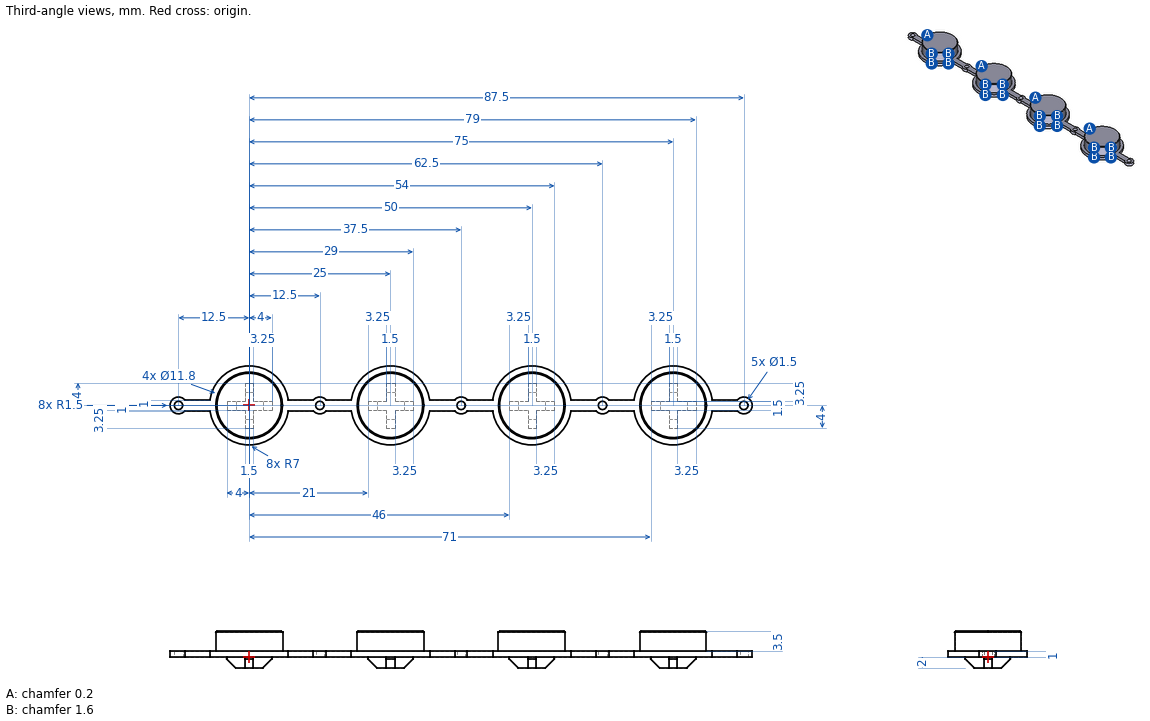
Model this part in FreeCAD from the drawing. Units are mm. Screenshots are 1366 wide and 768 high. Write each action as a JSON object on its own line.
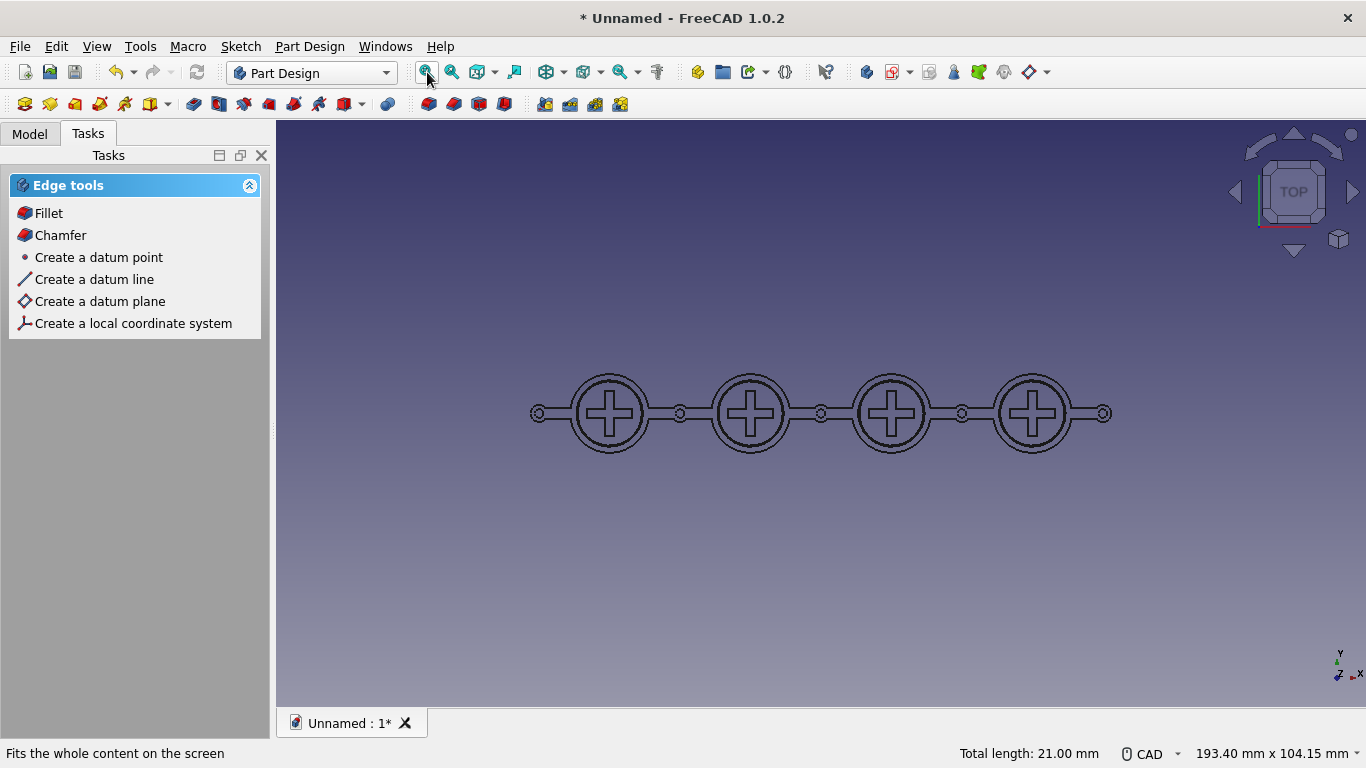
{"action": "key", "text": "1"}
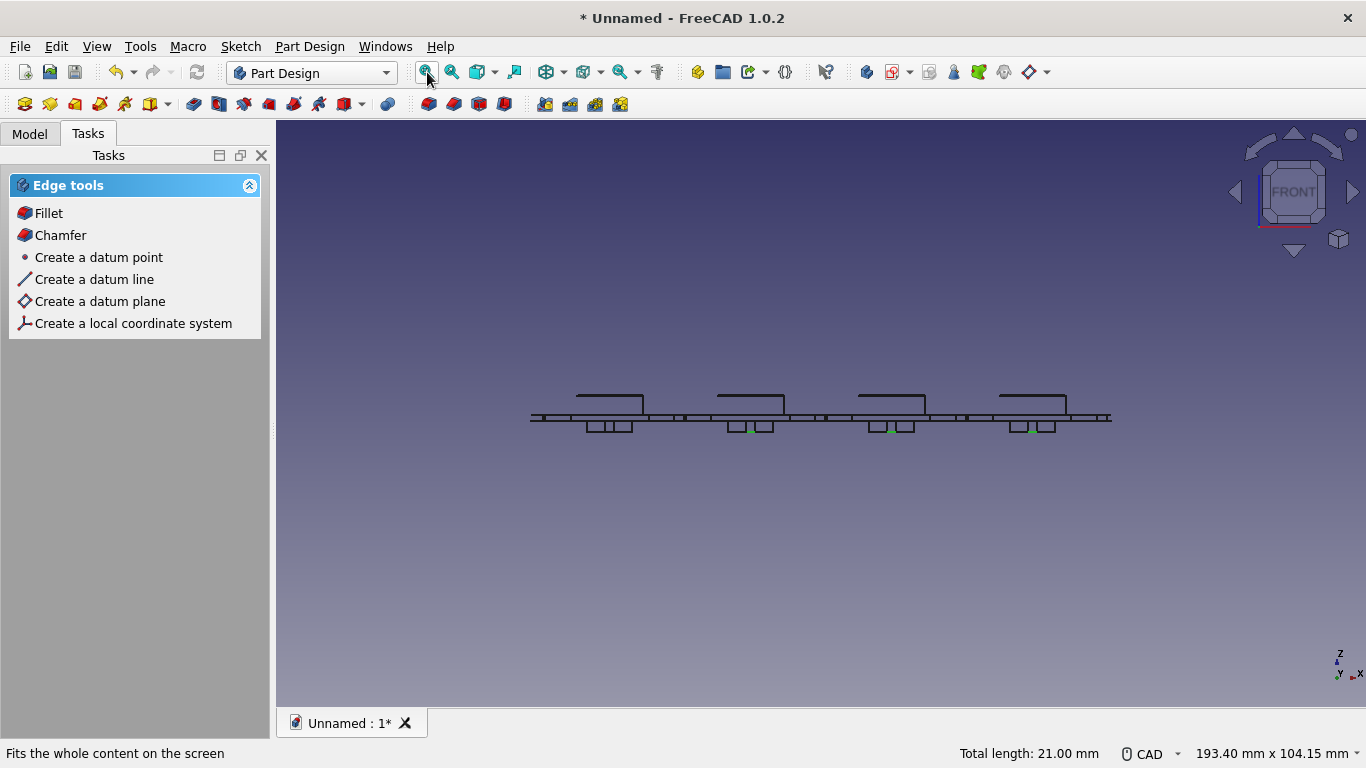
{"action": "scroll", "coordinate": [610, 431], "scroll_direction": "up", "scroll_amount": 8}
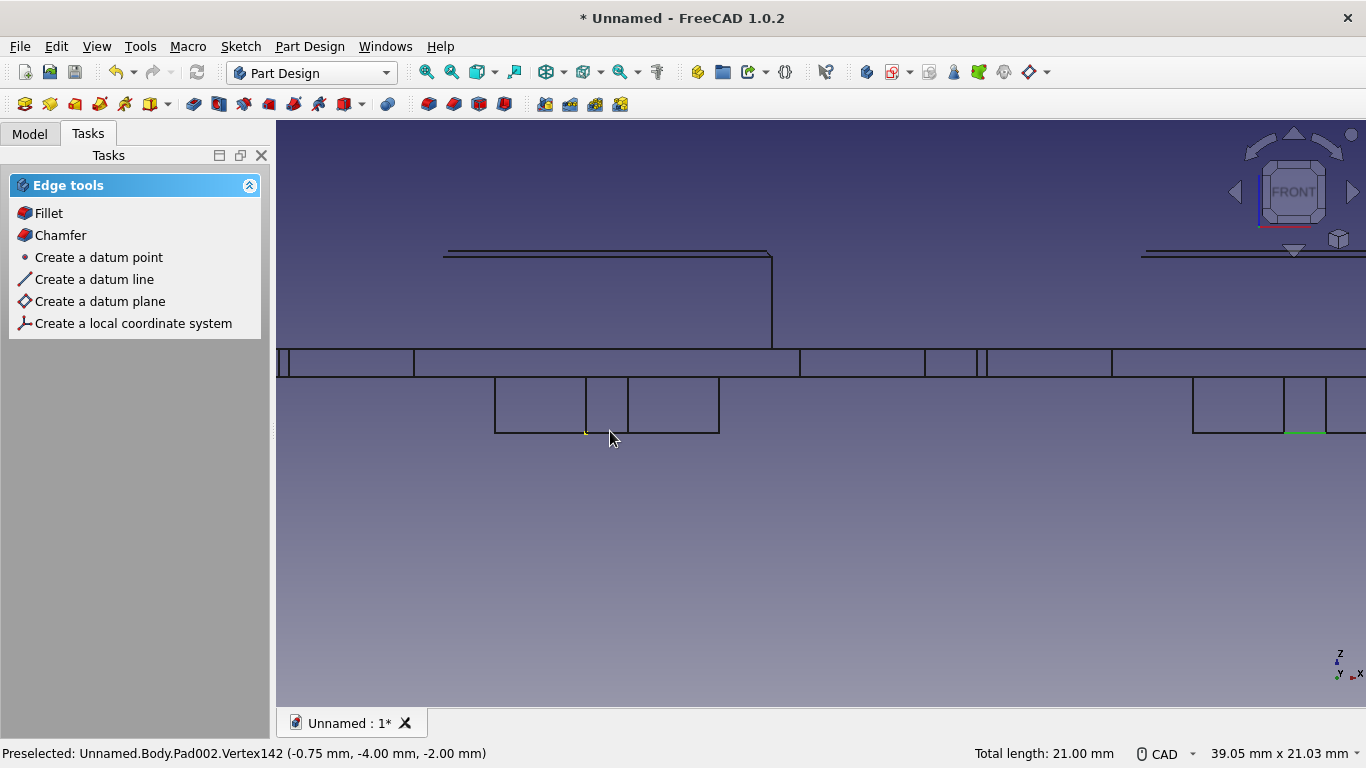
{"action": "left_click", "coordinate": [607, 432], "text": "ctrl"}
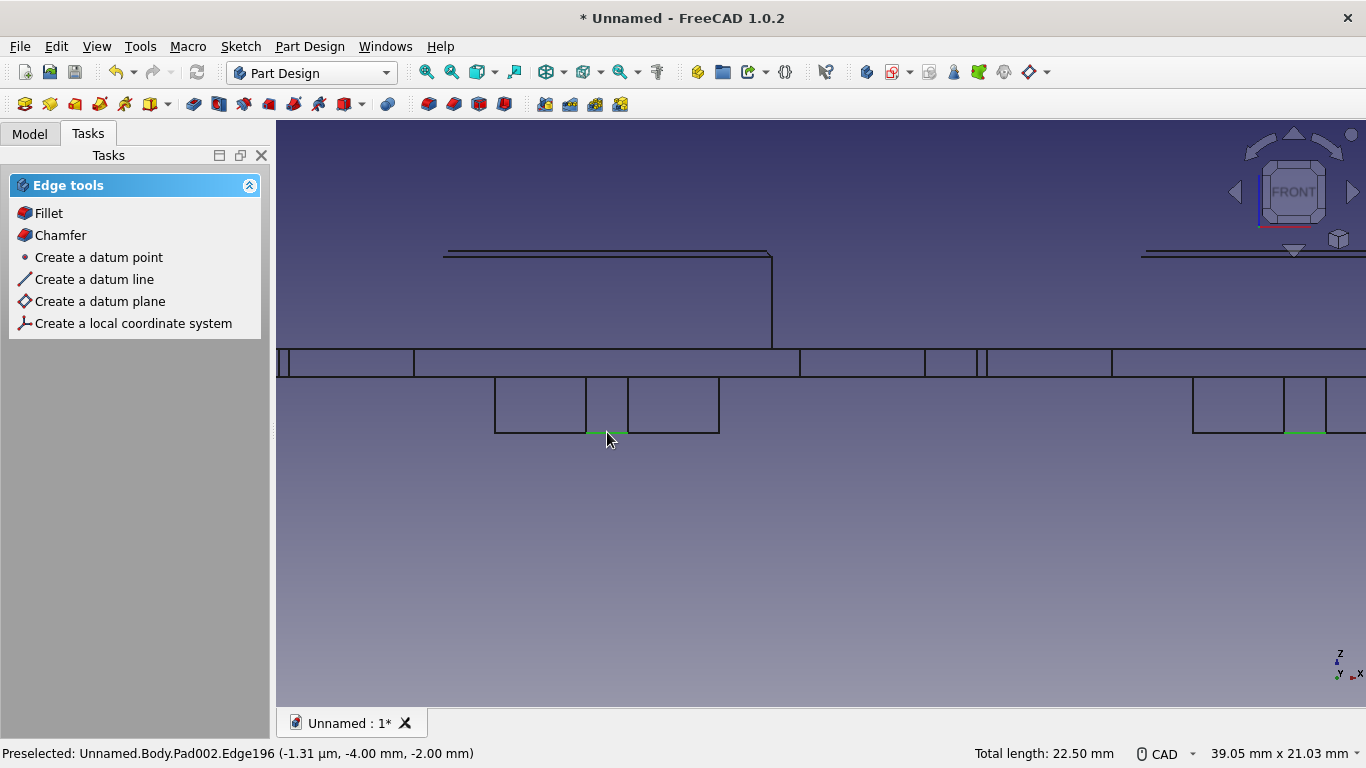
{"action": "key", "text": "v f"}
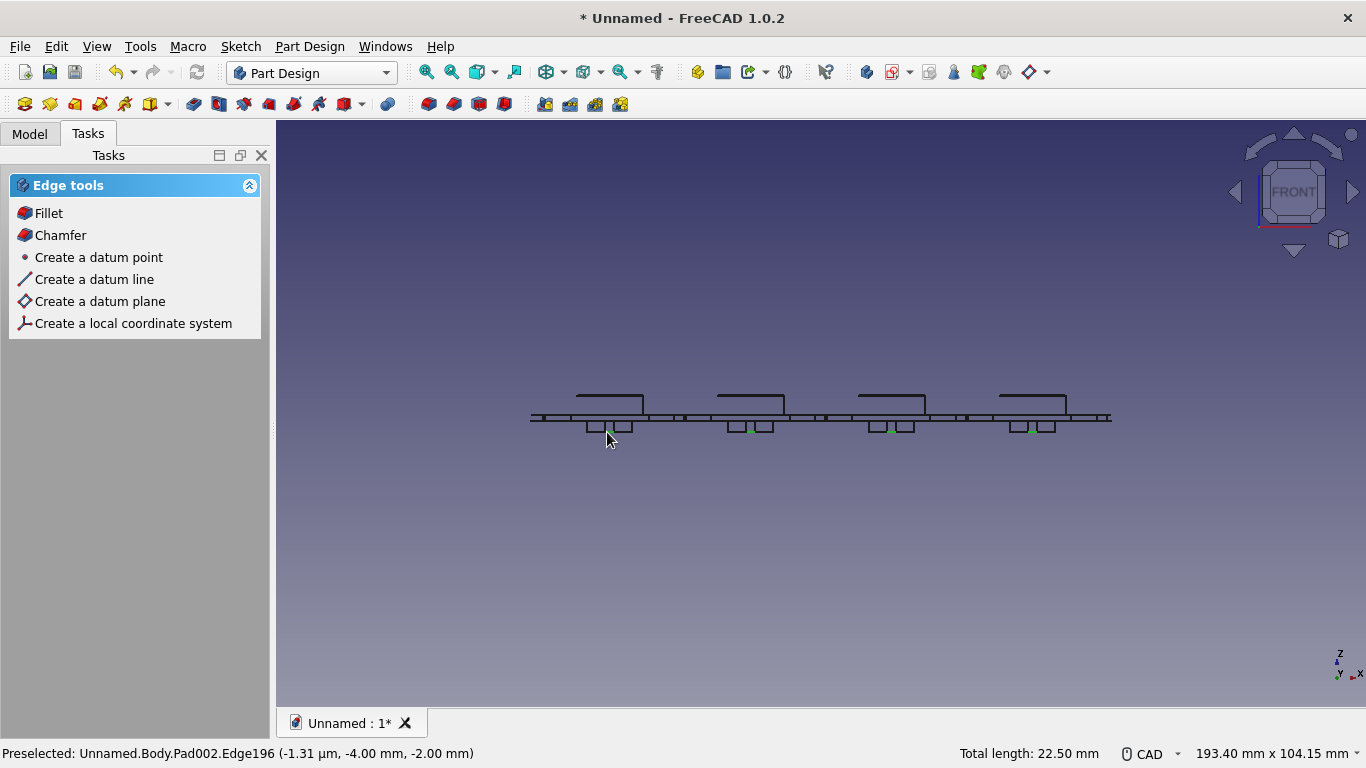
{"action": "key", "text": "3"}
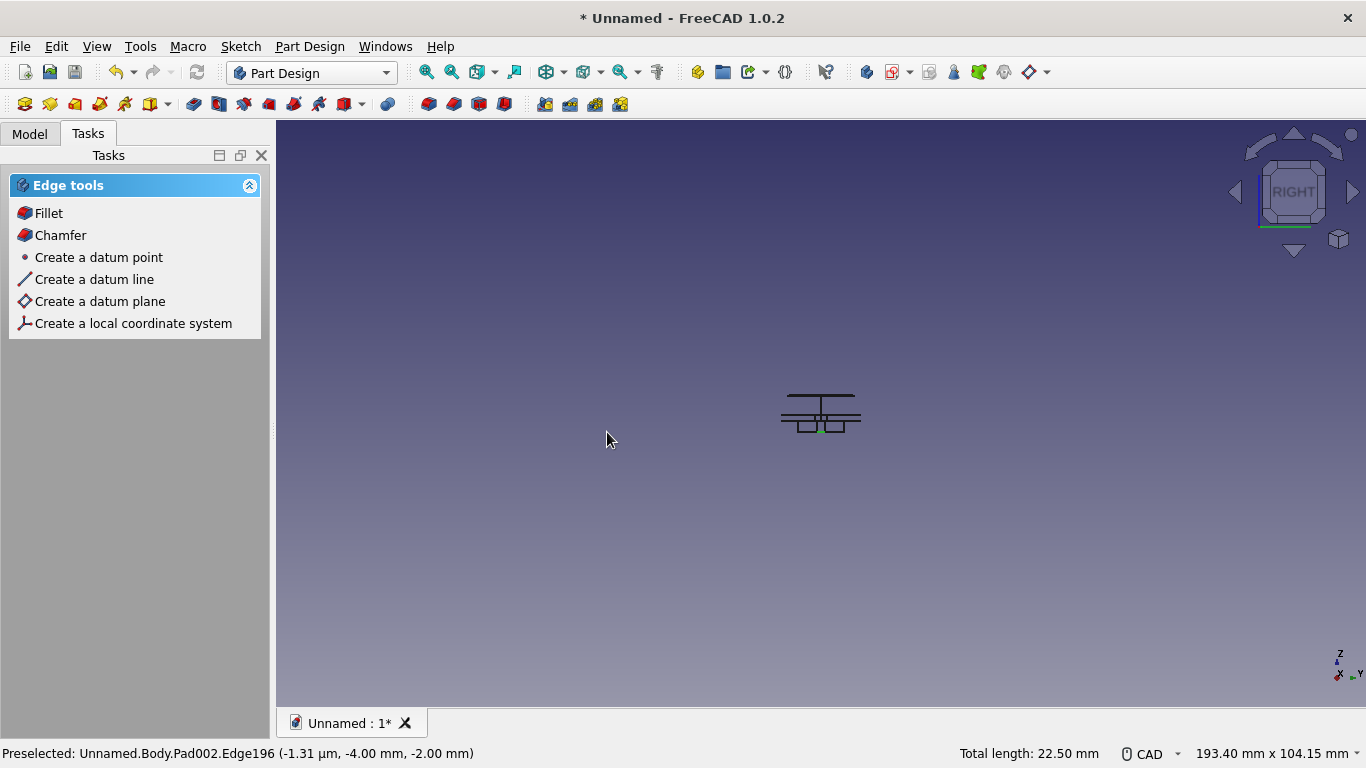
{"action": "key", "text": "v f"}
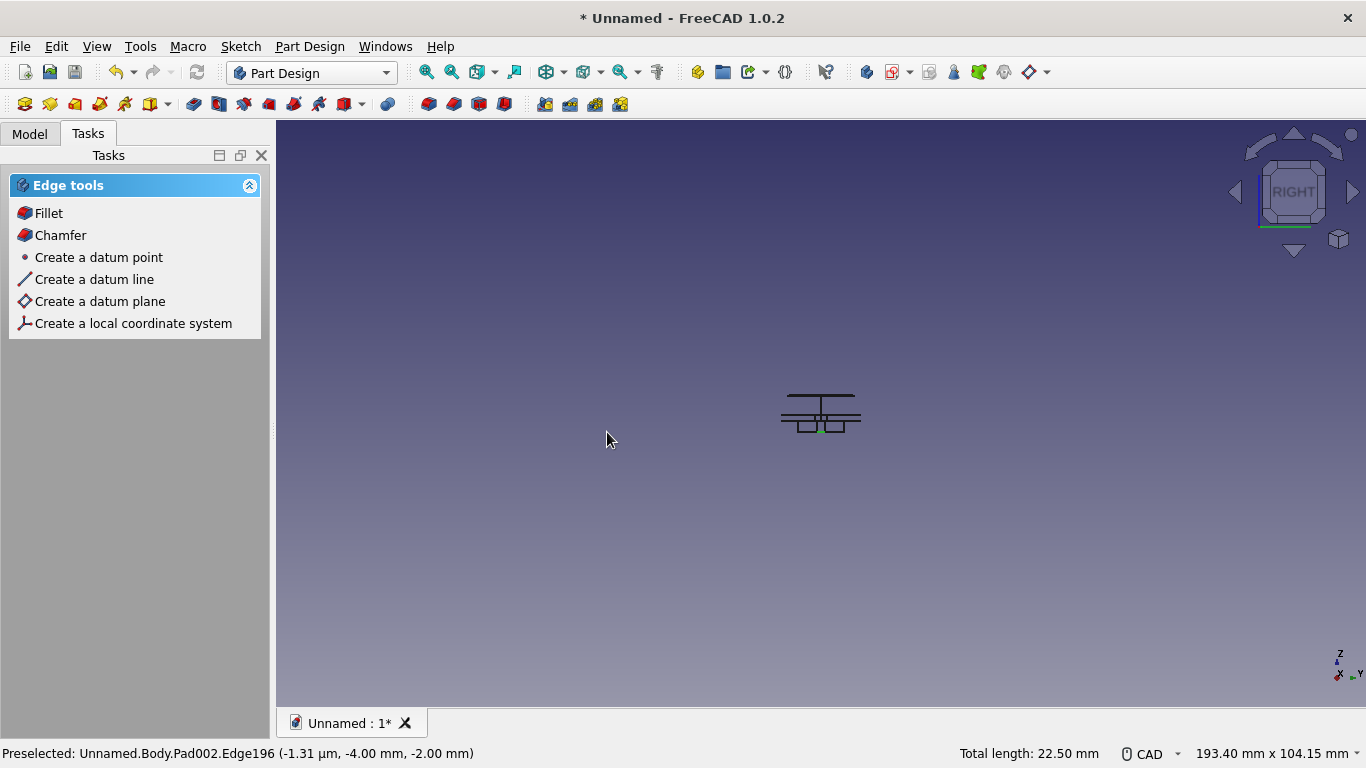
{"action": "scroll", "coordinate": [844, 431], "scroll_direction": "up", "scroll_amount": 8}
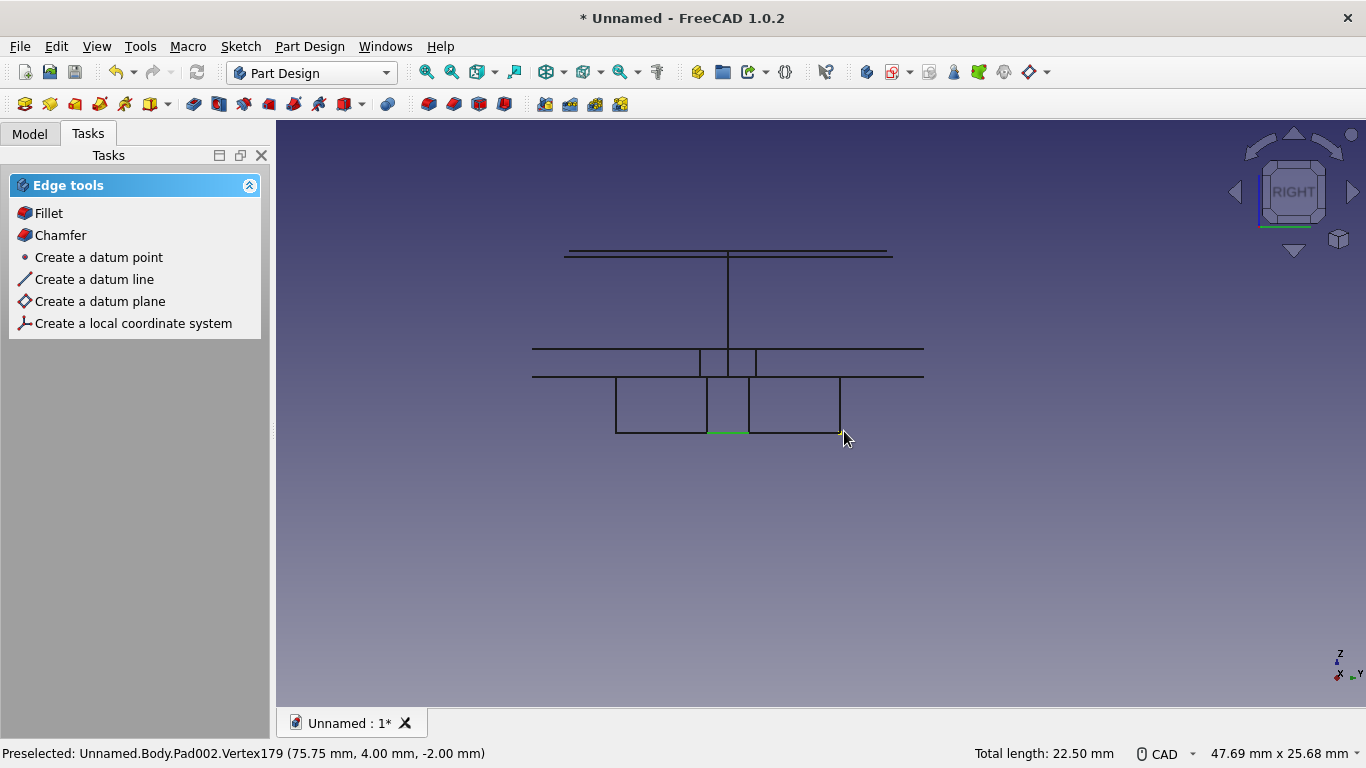
{"action": "key", "text": "v f"}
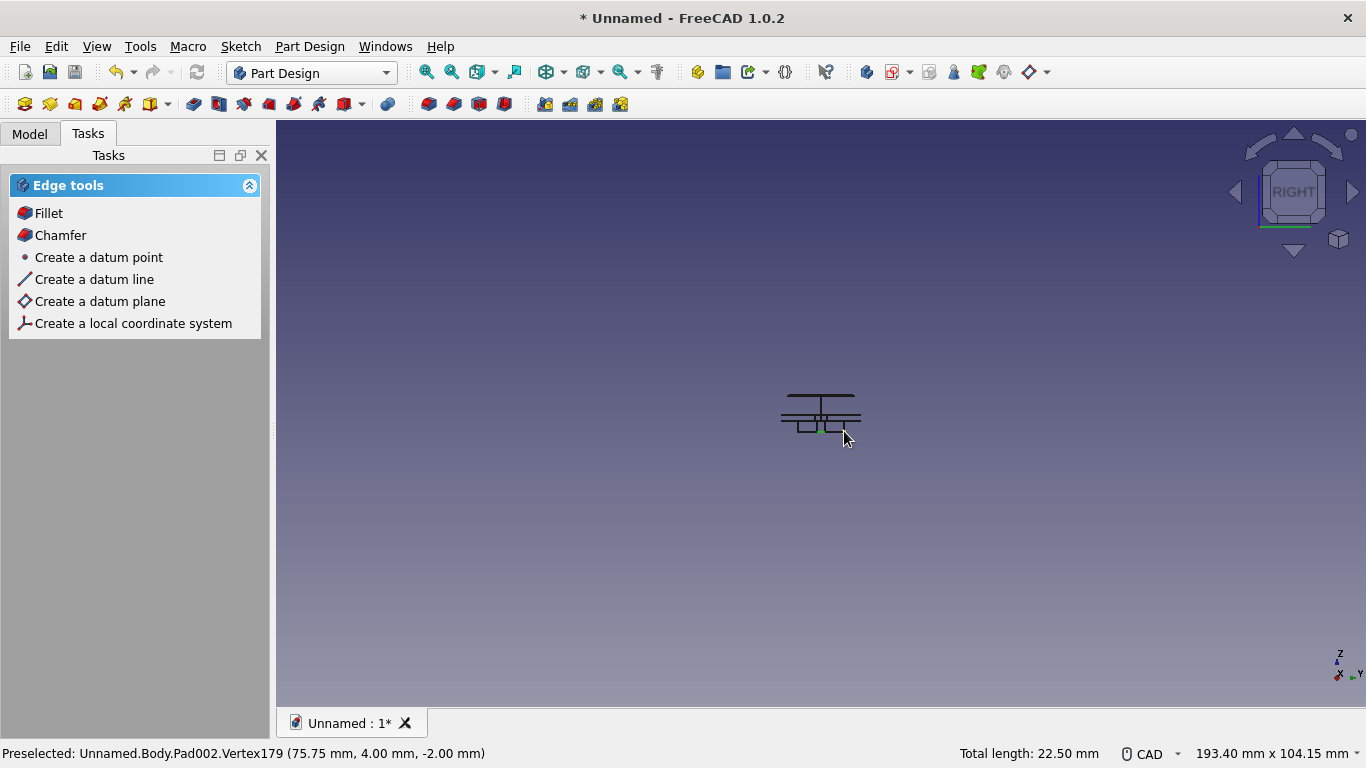
{"action": "key", "text": "5"}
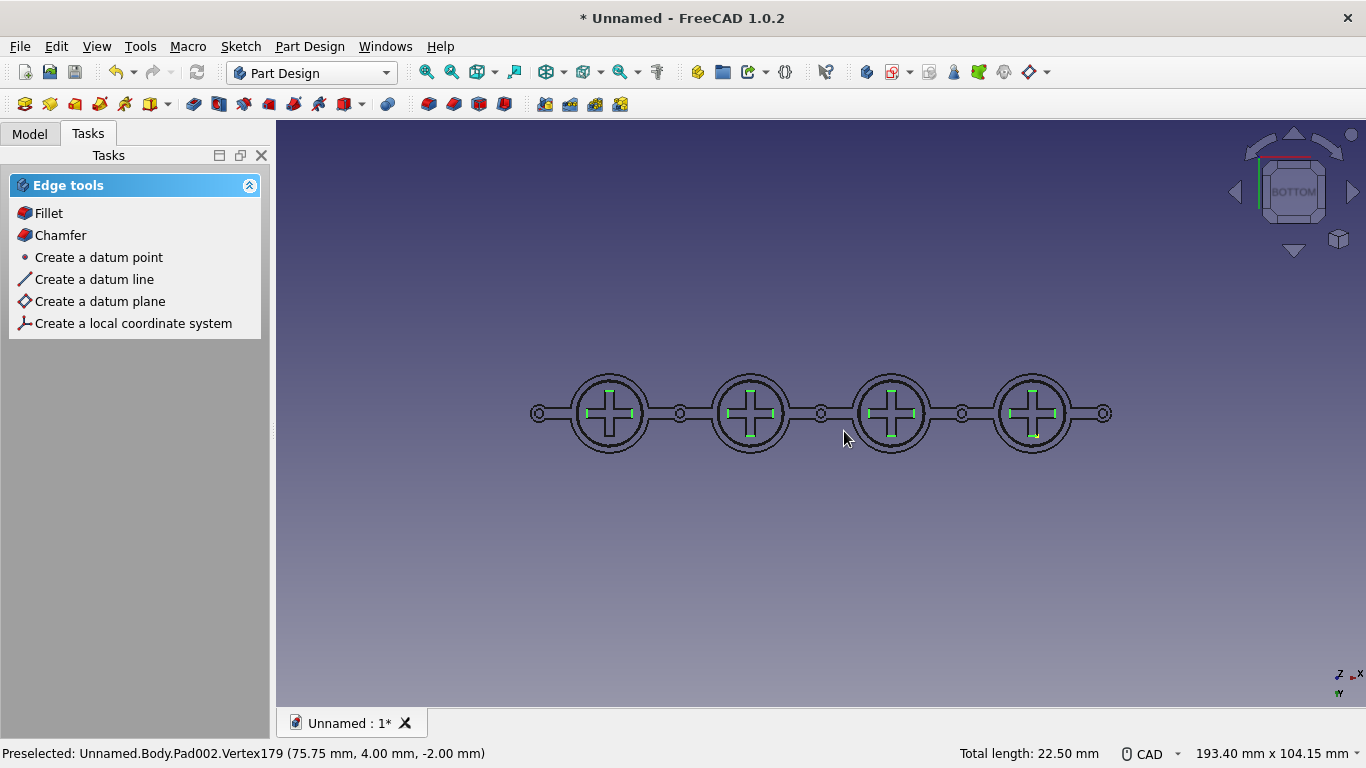
{"action": "scroll", "coordinate": [610, 435], "scroll_direction": "up", "scroll_amount": 8}